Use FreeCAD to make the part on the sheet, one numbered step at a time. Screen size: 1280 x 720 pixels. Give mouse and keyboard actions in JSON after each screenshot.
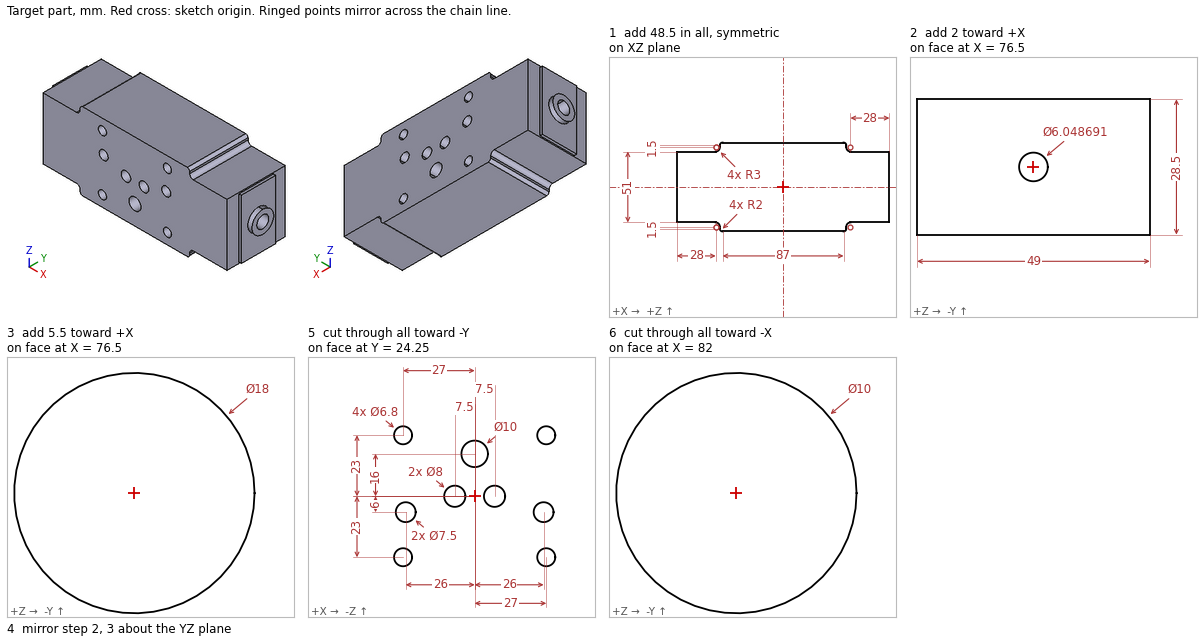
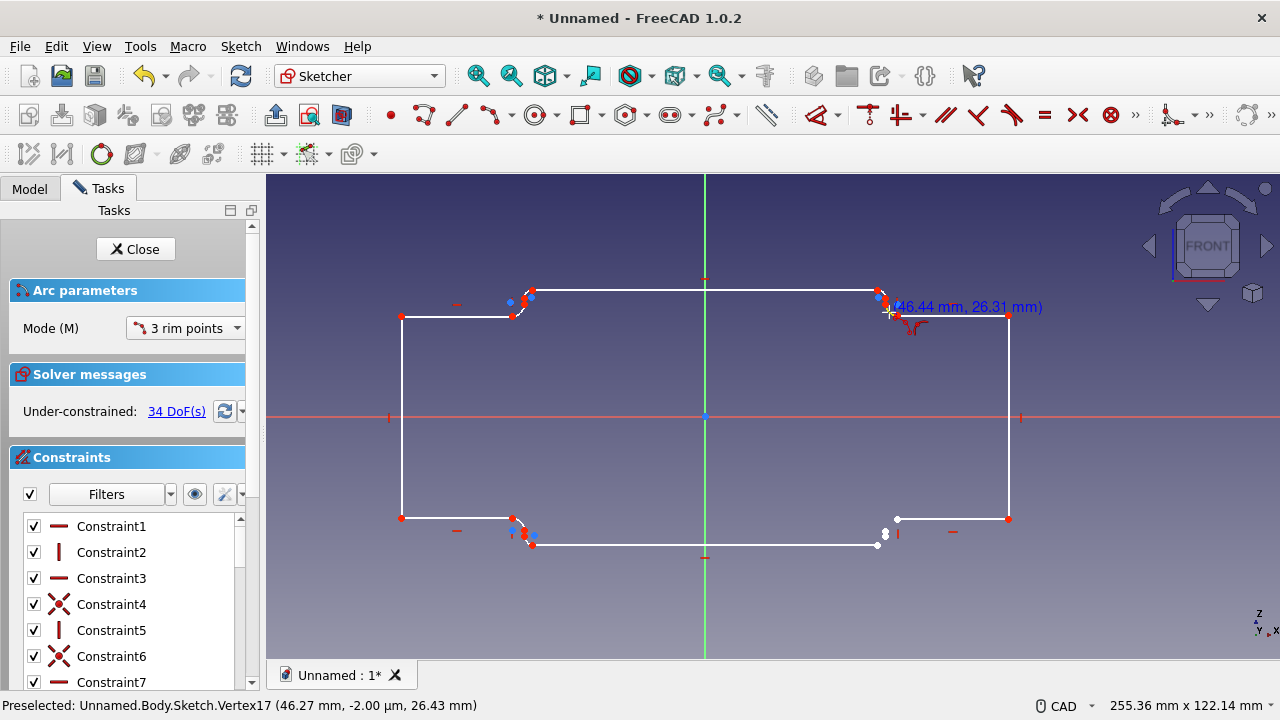
{"action": "left_click", "coordinate": [898, 519]}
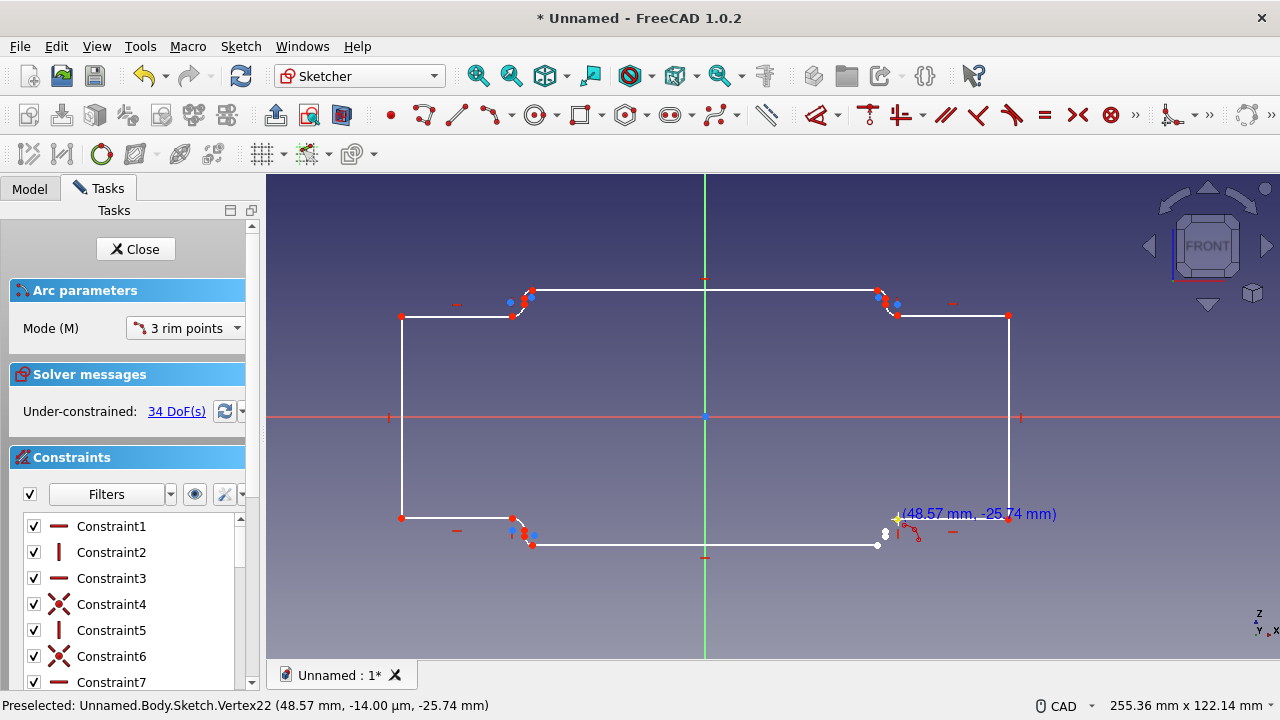
{"action": "scroll", "coordinate": [886, 530], "scroll_direction": "up", "scroll_amount": 9}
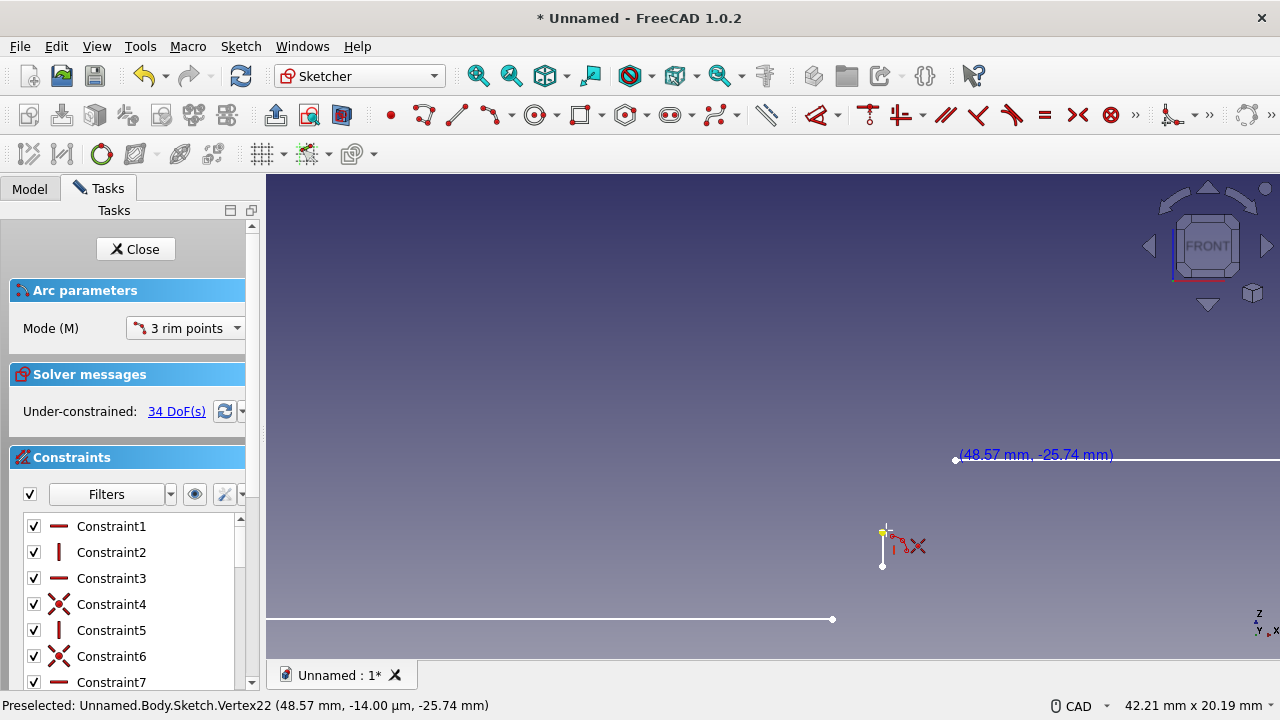
{"action": "left_click", "coordinate": [883, 533]}
{"action": "left_click", "coordinate": [903, 476]}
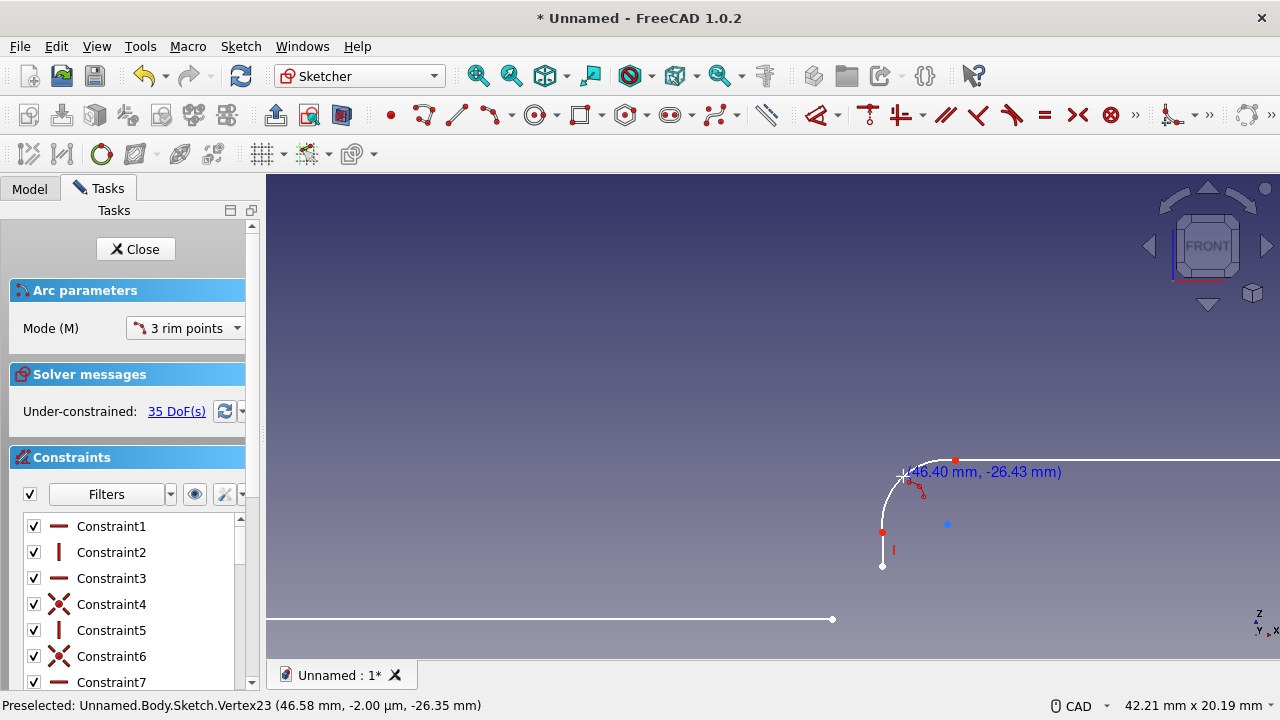
{"action": "left_click", "coordinate": [883, 566]}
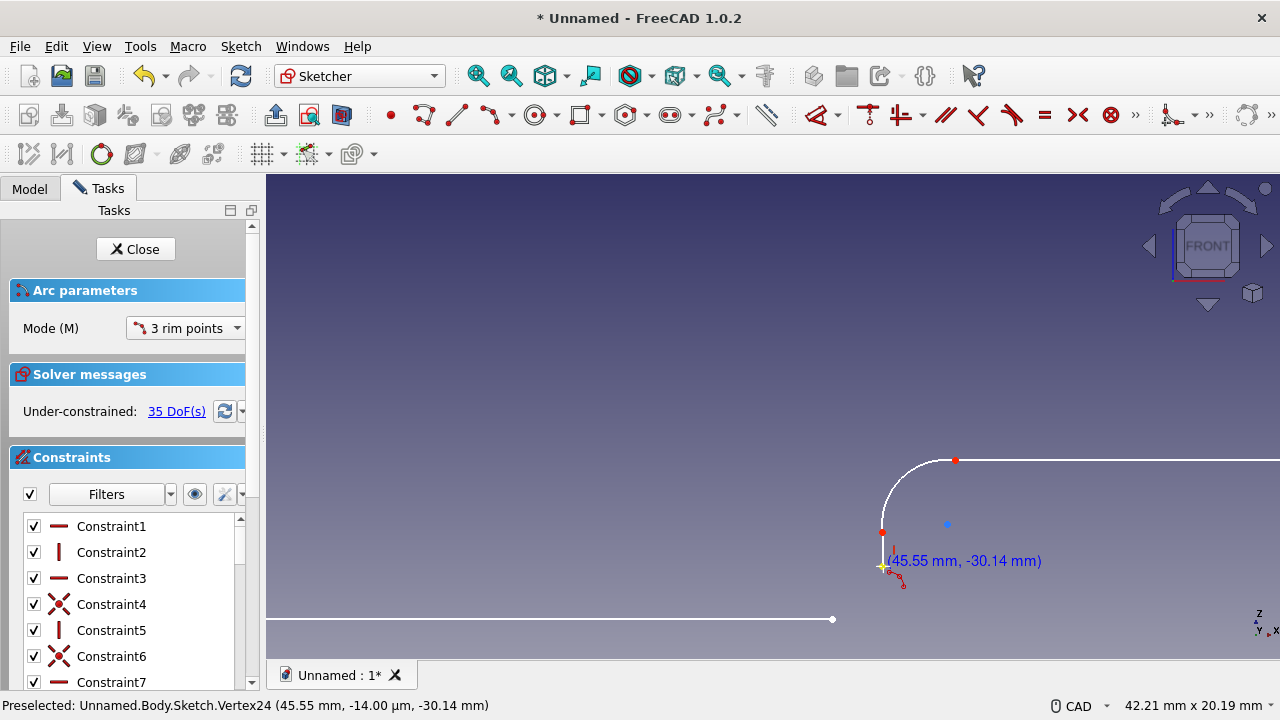
{"action": "scroll", "coordinate": [886, 530], "scroll_direction": "down", "scroll_amount": 9}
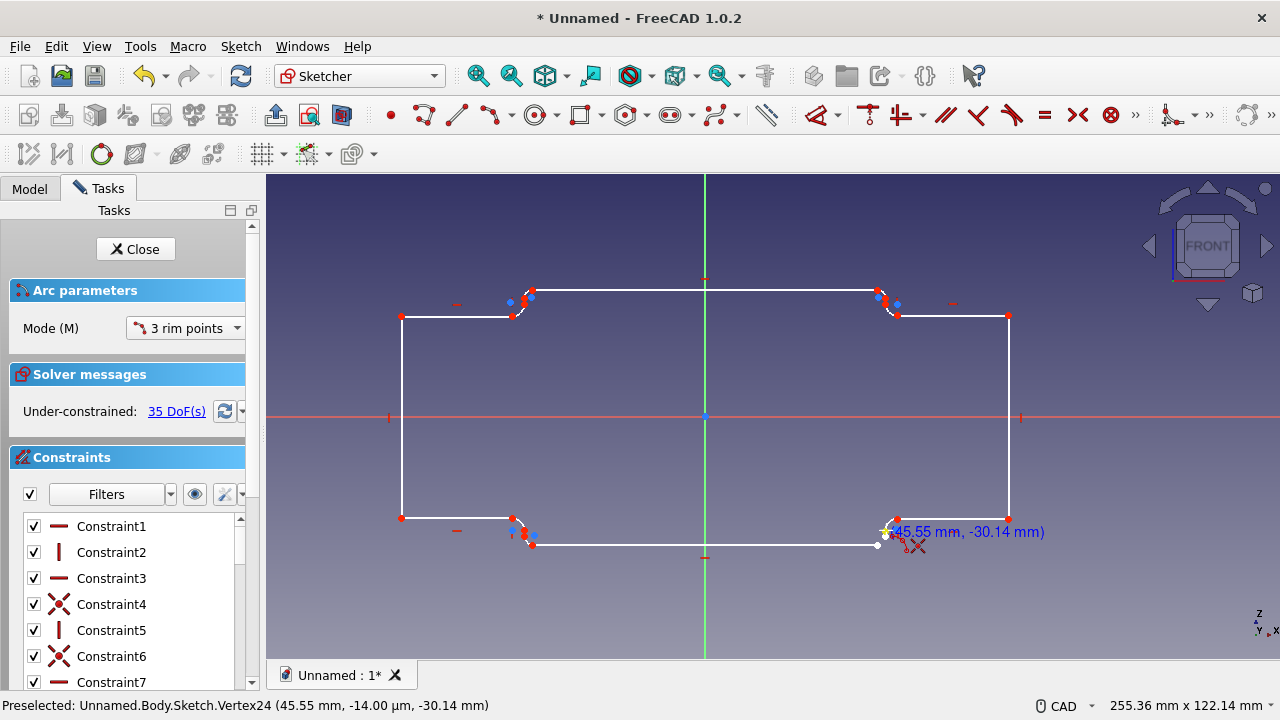
{"action": "scroll", "coordinate": [878, 544], "scroll_direction": "up", "scroll_amount": 2}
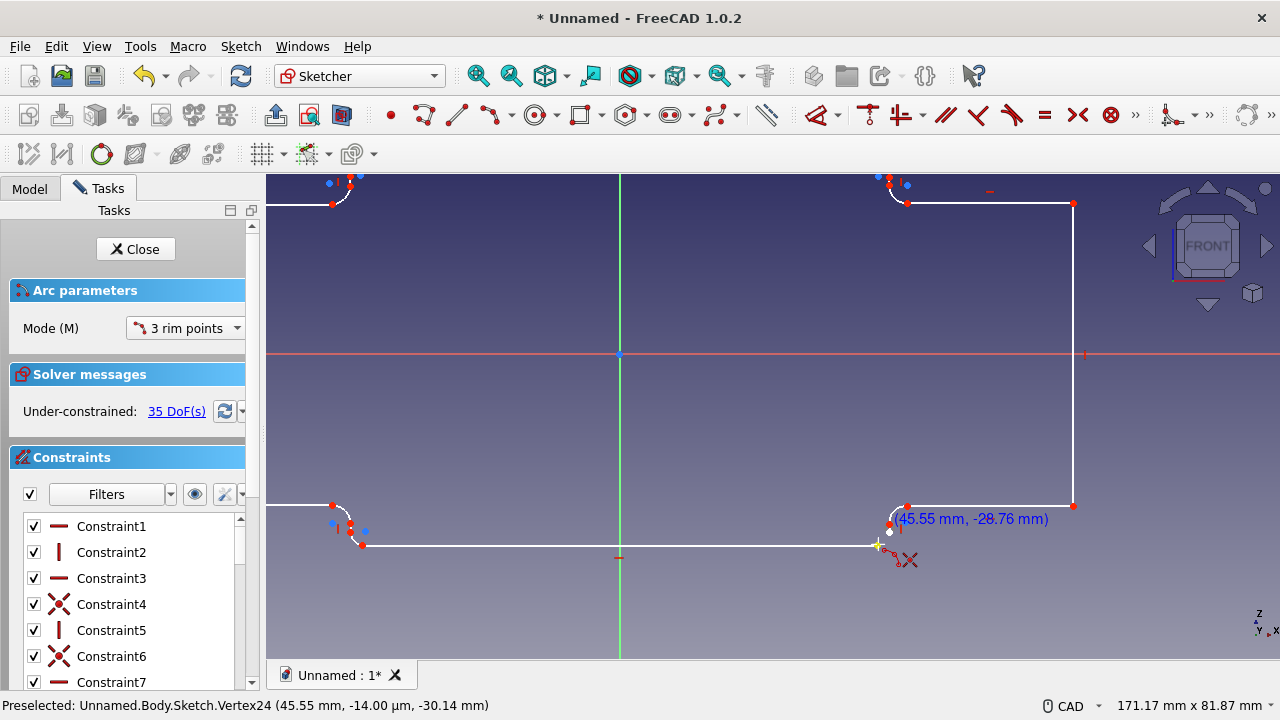
{"action": "left_click", "coordinate": [877, 546]}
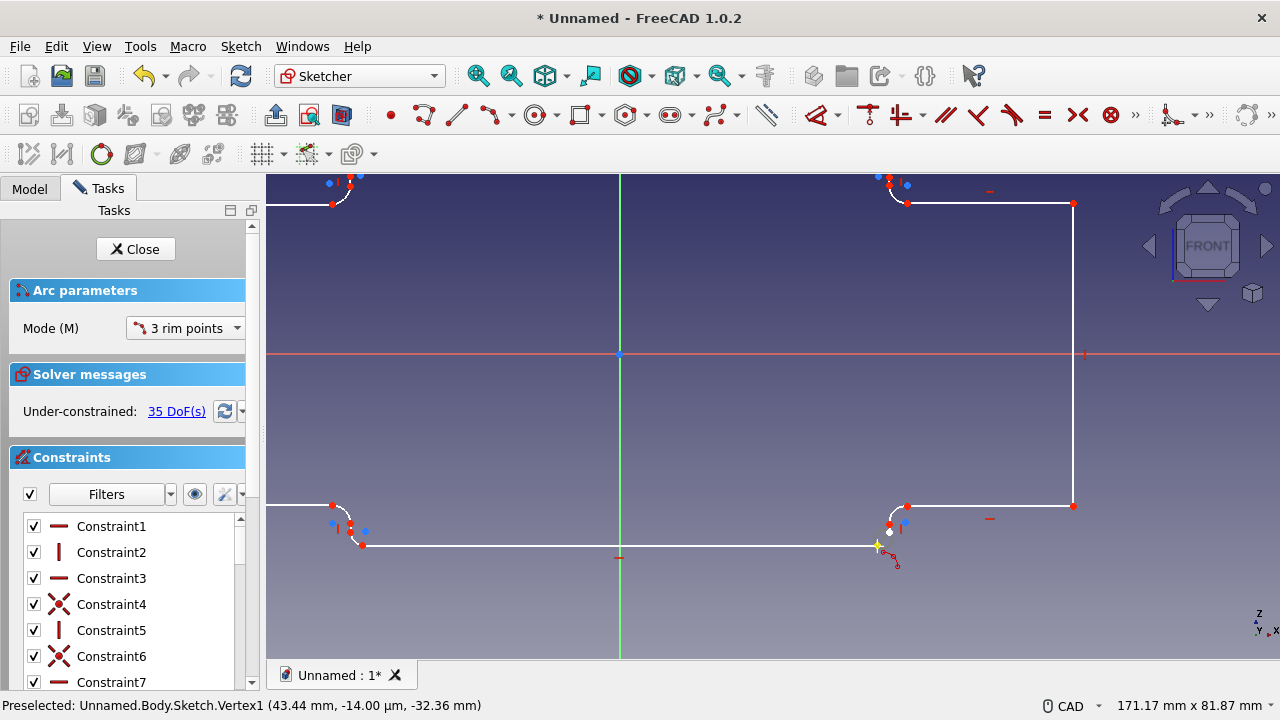
{"action": "scroll", "coordinate": [886, 540], "scroll_direction": "up", "scroll_amount": 8}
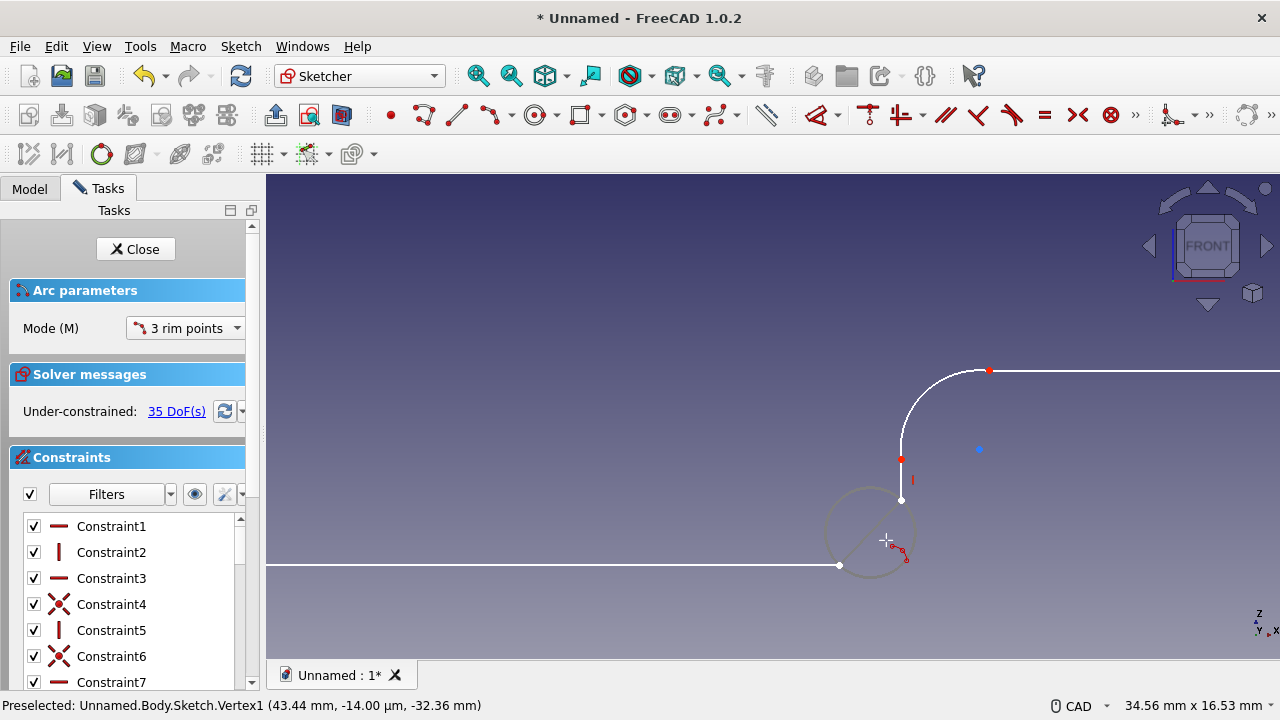
{"action": "left_click", "coordinate": [883, 538]}
{"action": "key", "text": "Escape"}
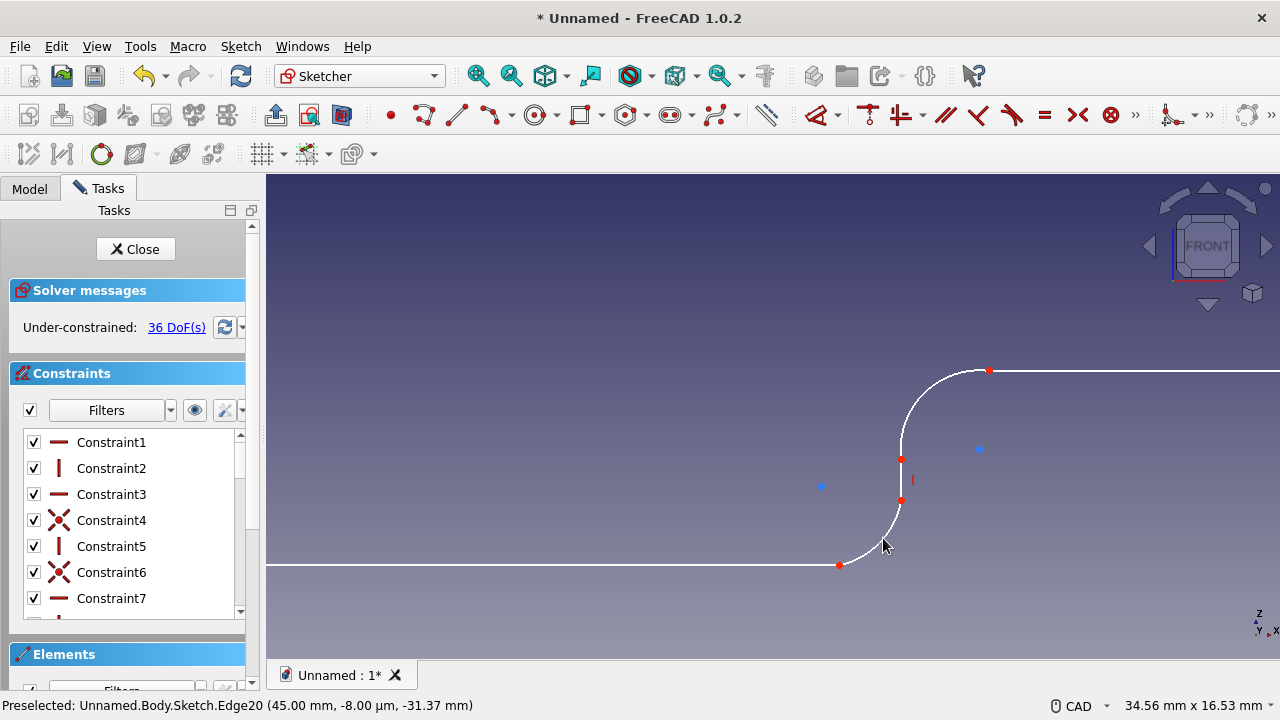
{"action": "scroll", "coordinate": [883, 542], "scroll_direction": "down", "scroll_amount": 10}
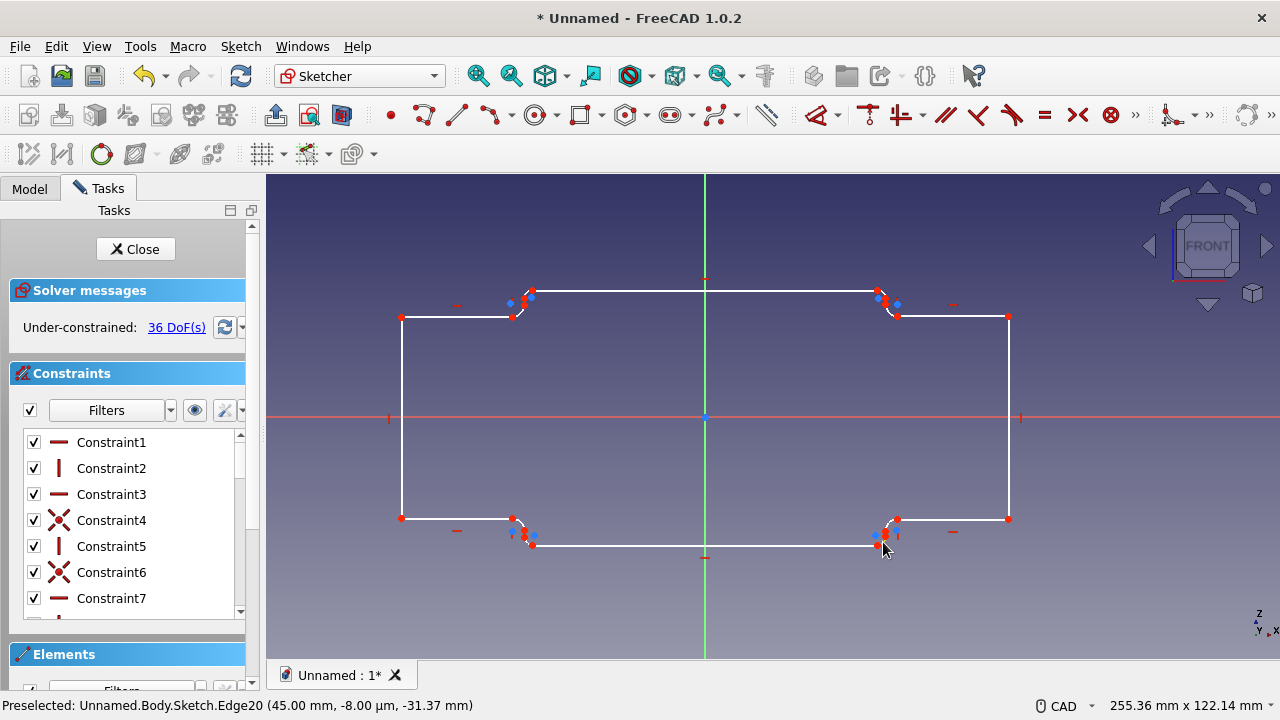
{"action": "left_click", "coordinate": [809, 546]}